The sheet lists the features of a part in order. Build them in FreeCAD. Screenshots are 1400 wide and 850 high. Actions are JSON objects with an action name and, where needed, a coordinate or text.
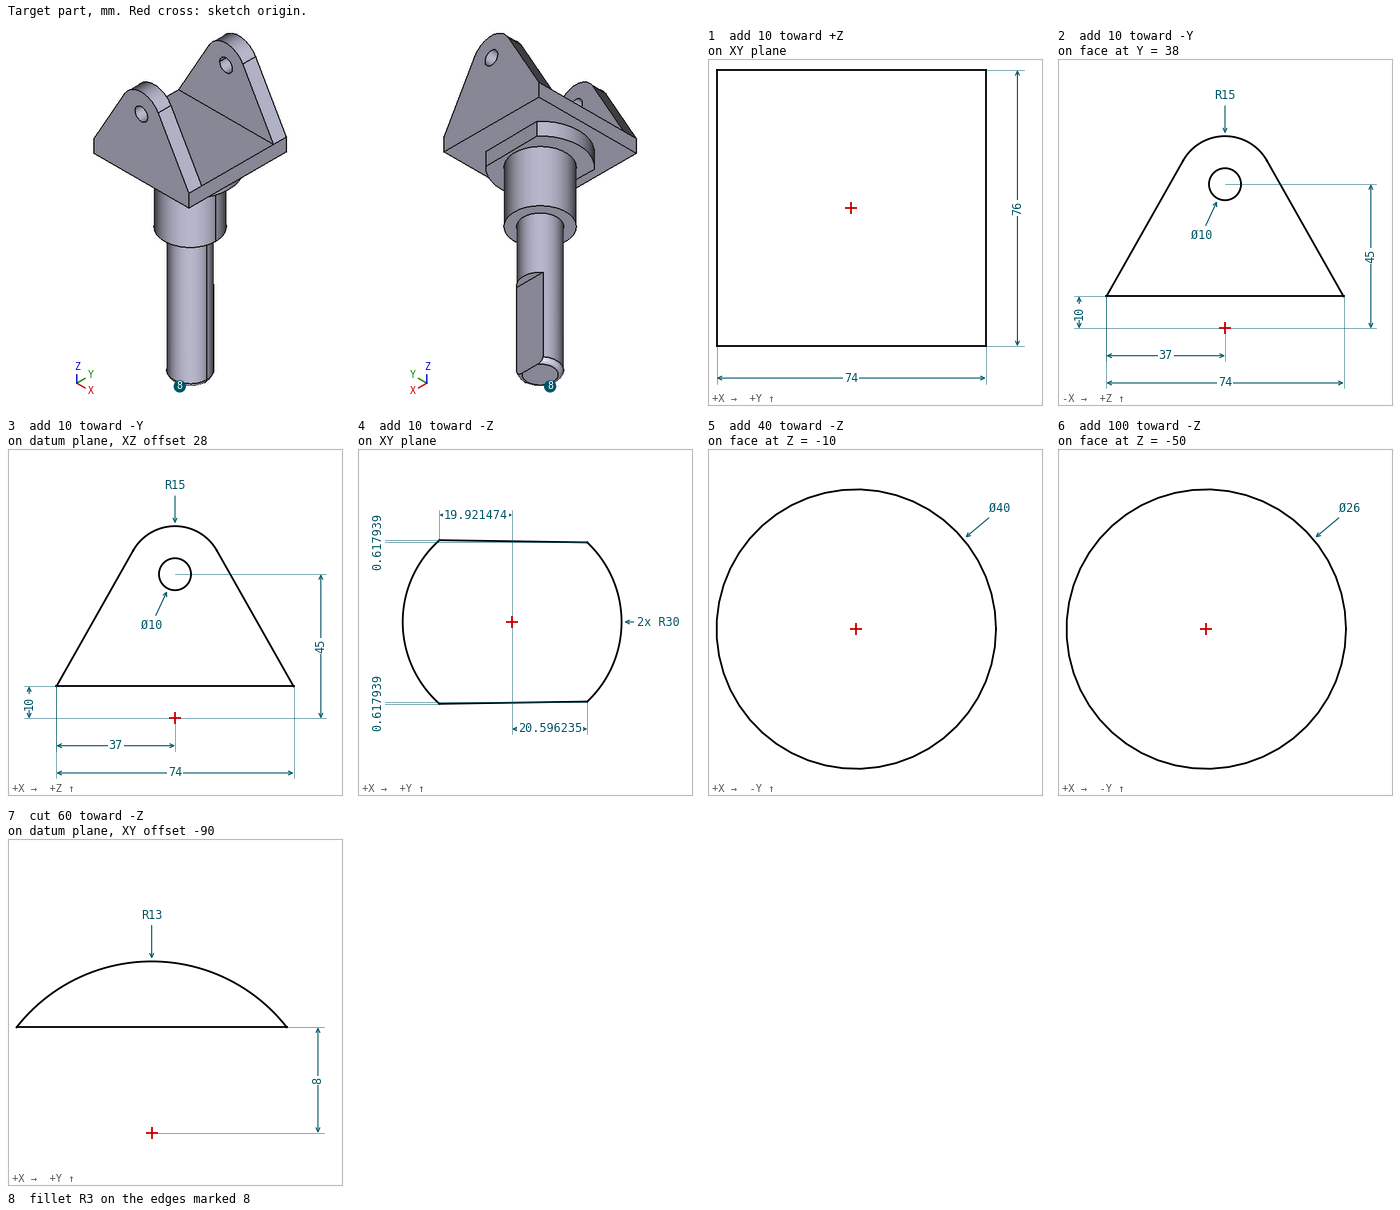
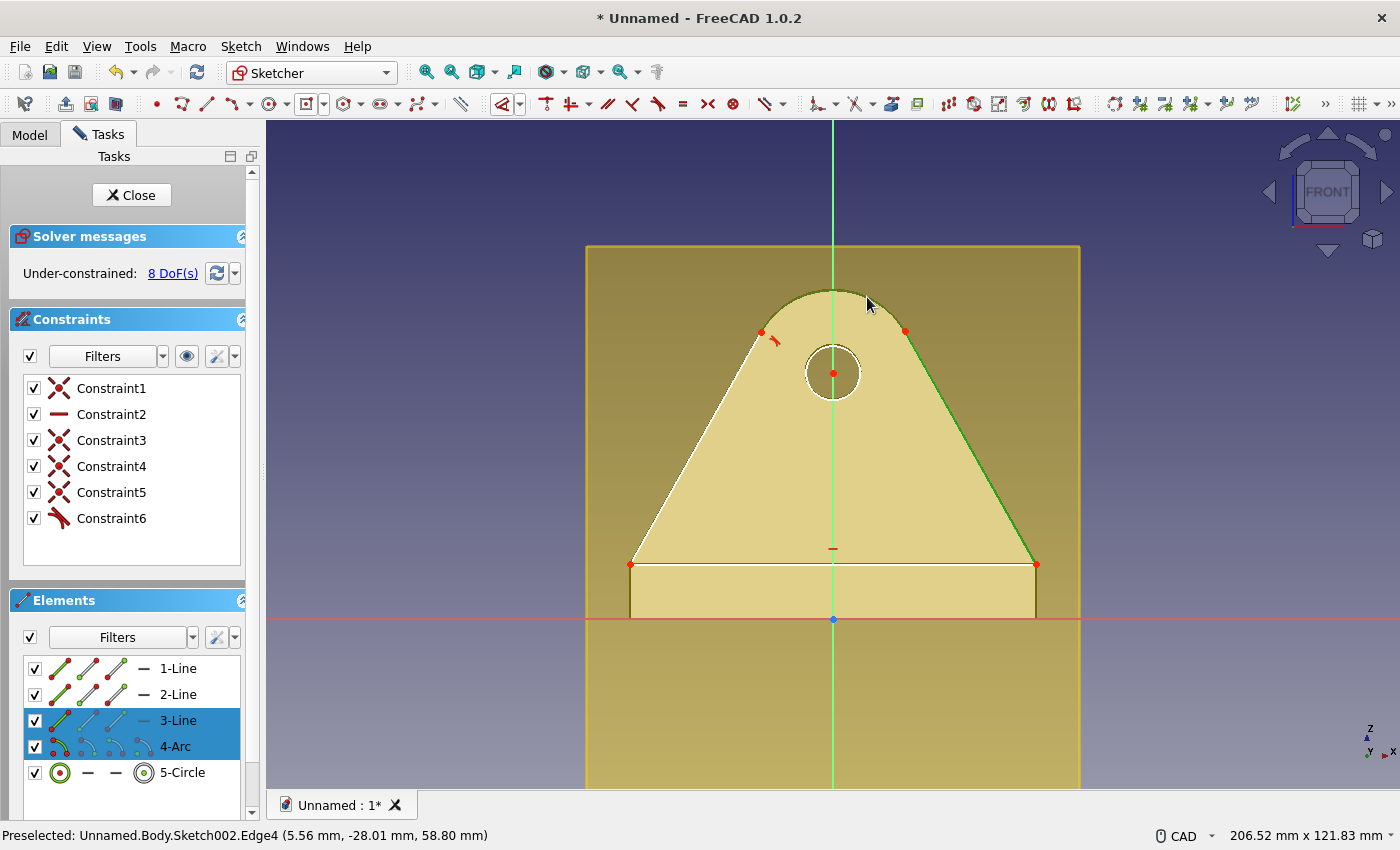
{"action": "left_click", "coordinate": [658, 104]}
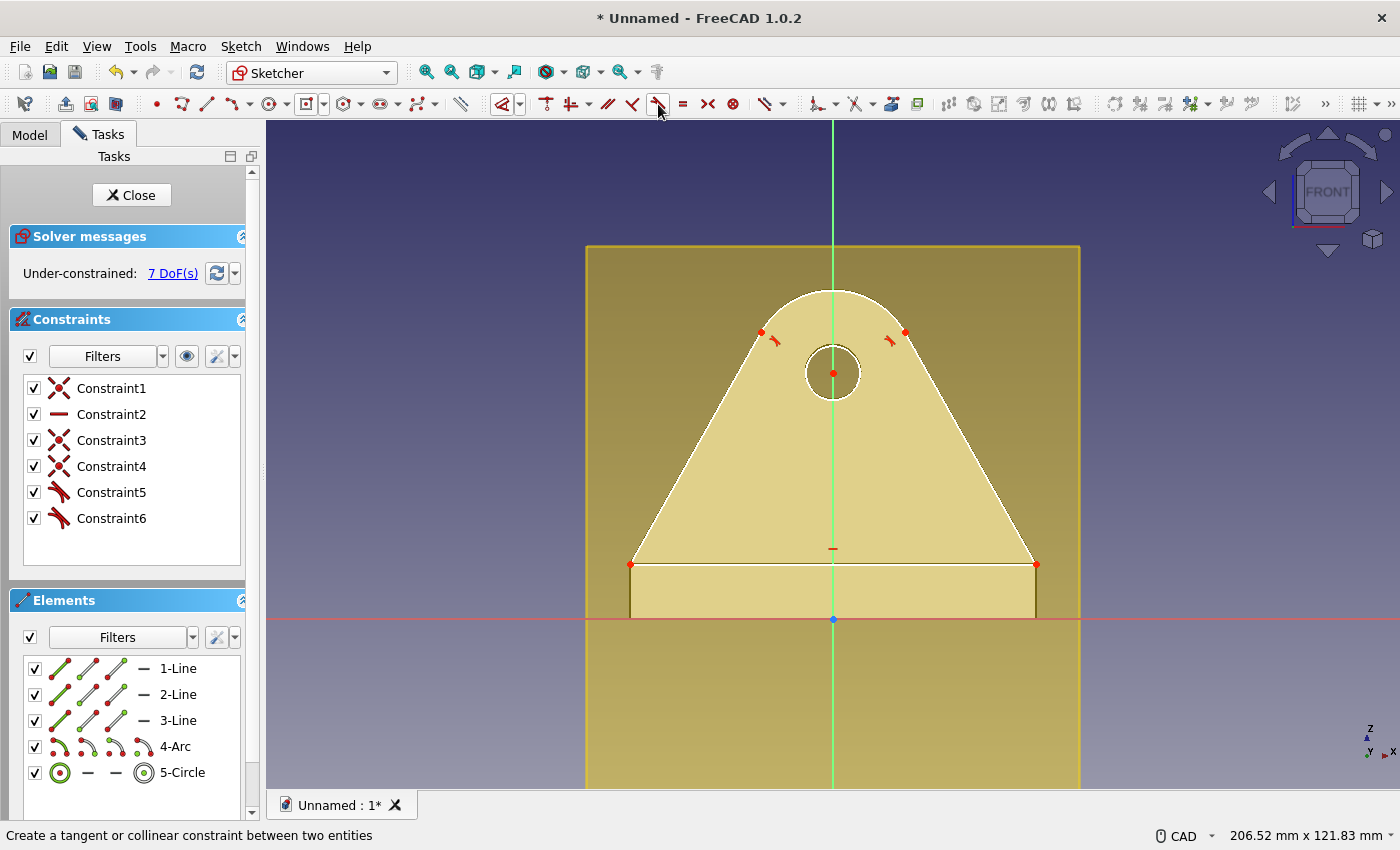
{"action": "left_click", "coordinate": [833, 373]}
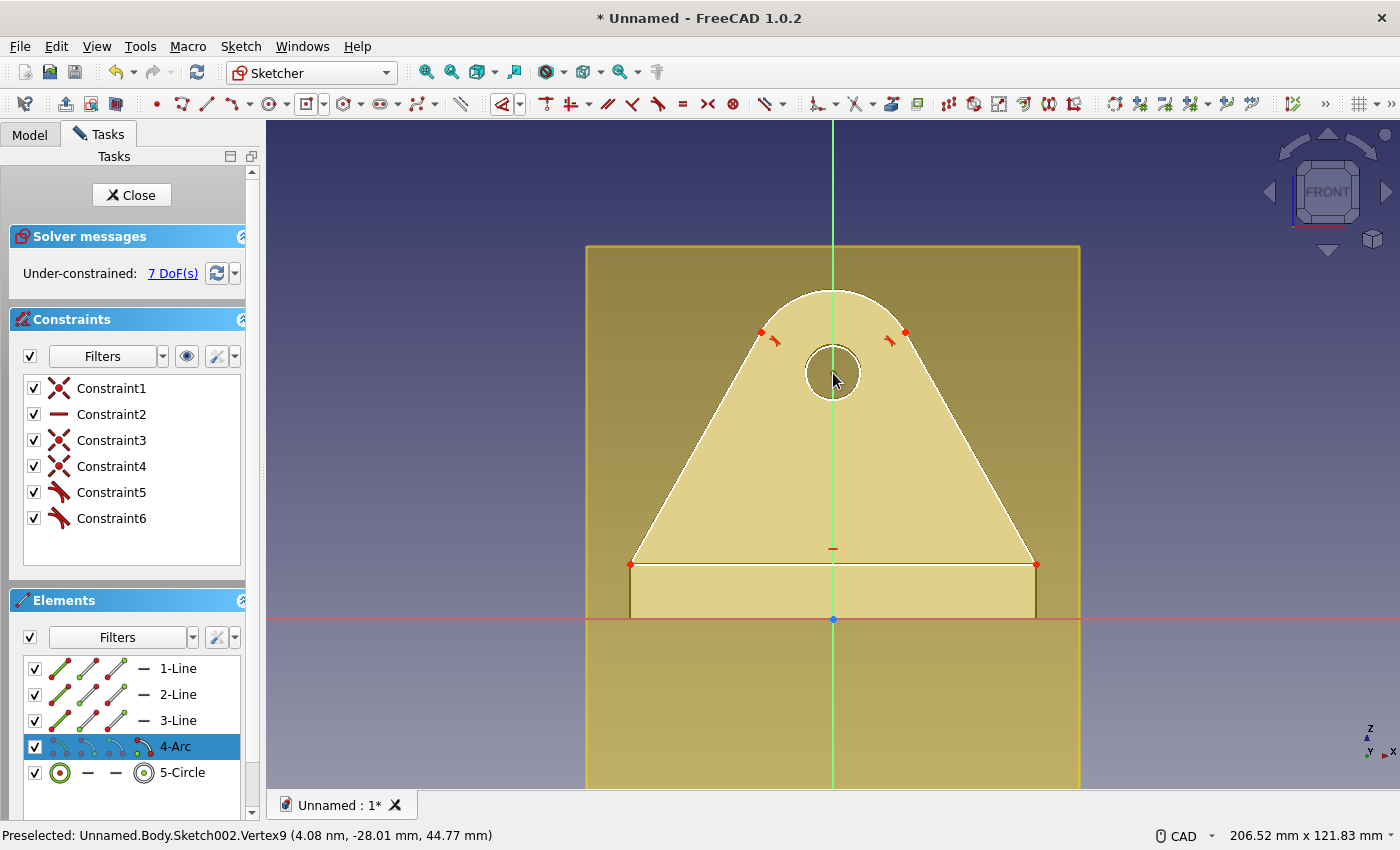
{"action": "left_click", "coordinate": [833, 717]}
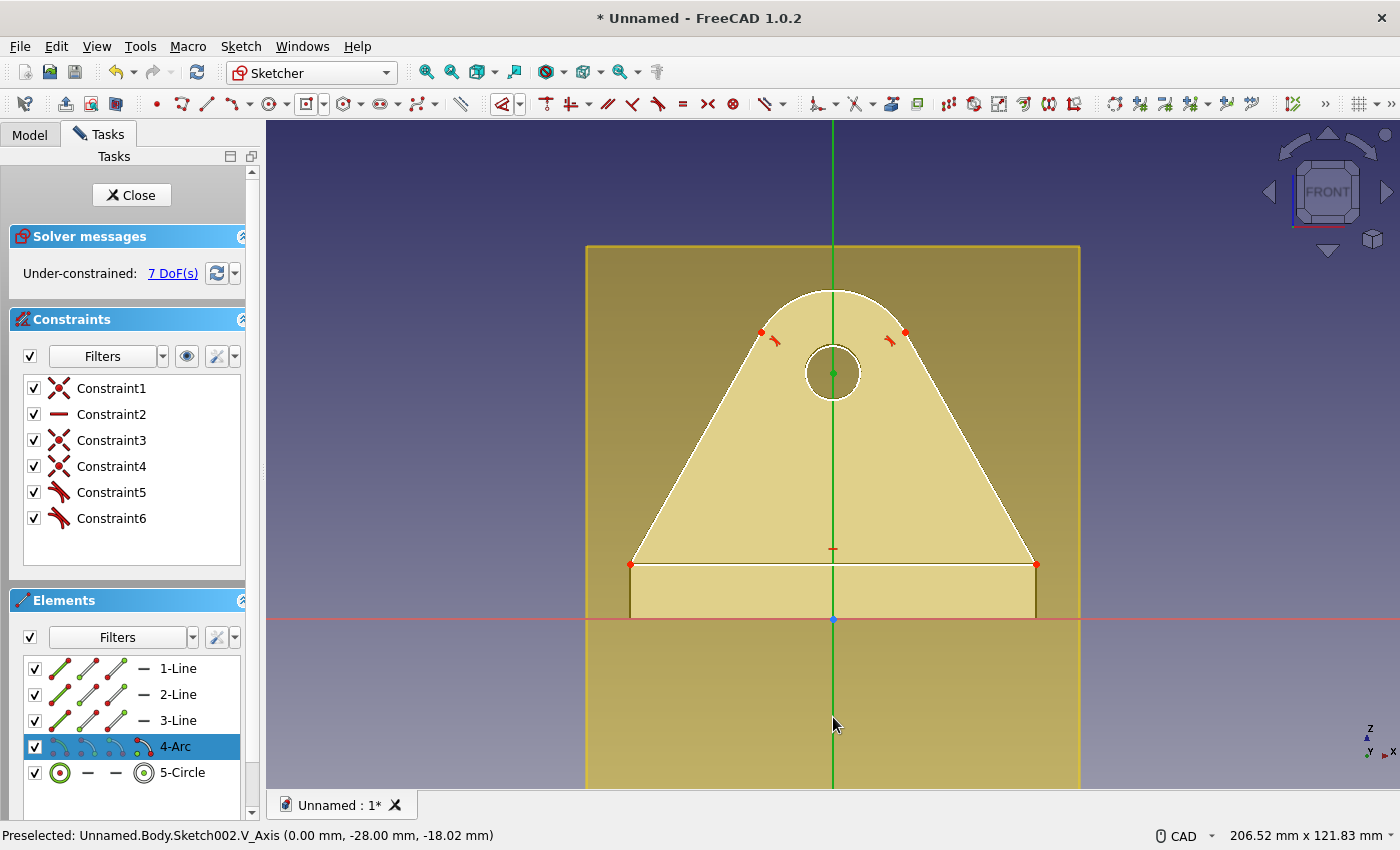
{"action": "left_click", "coordinate": [546, 104]}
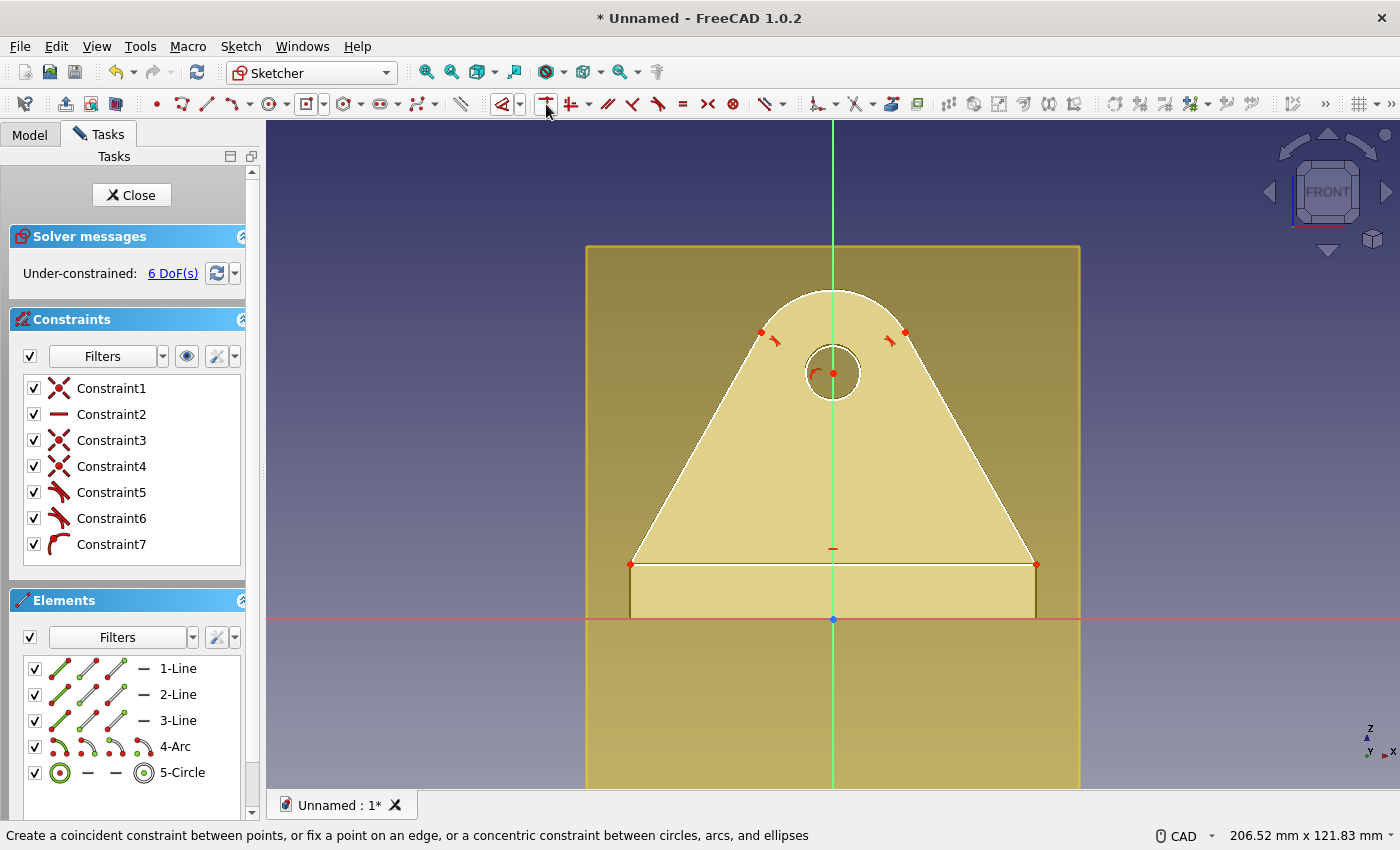
{"action": "left_click", "coordinate": [867, 298]}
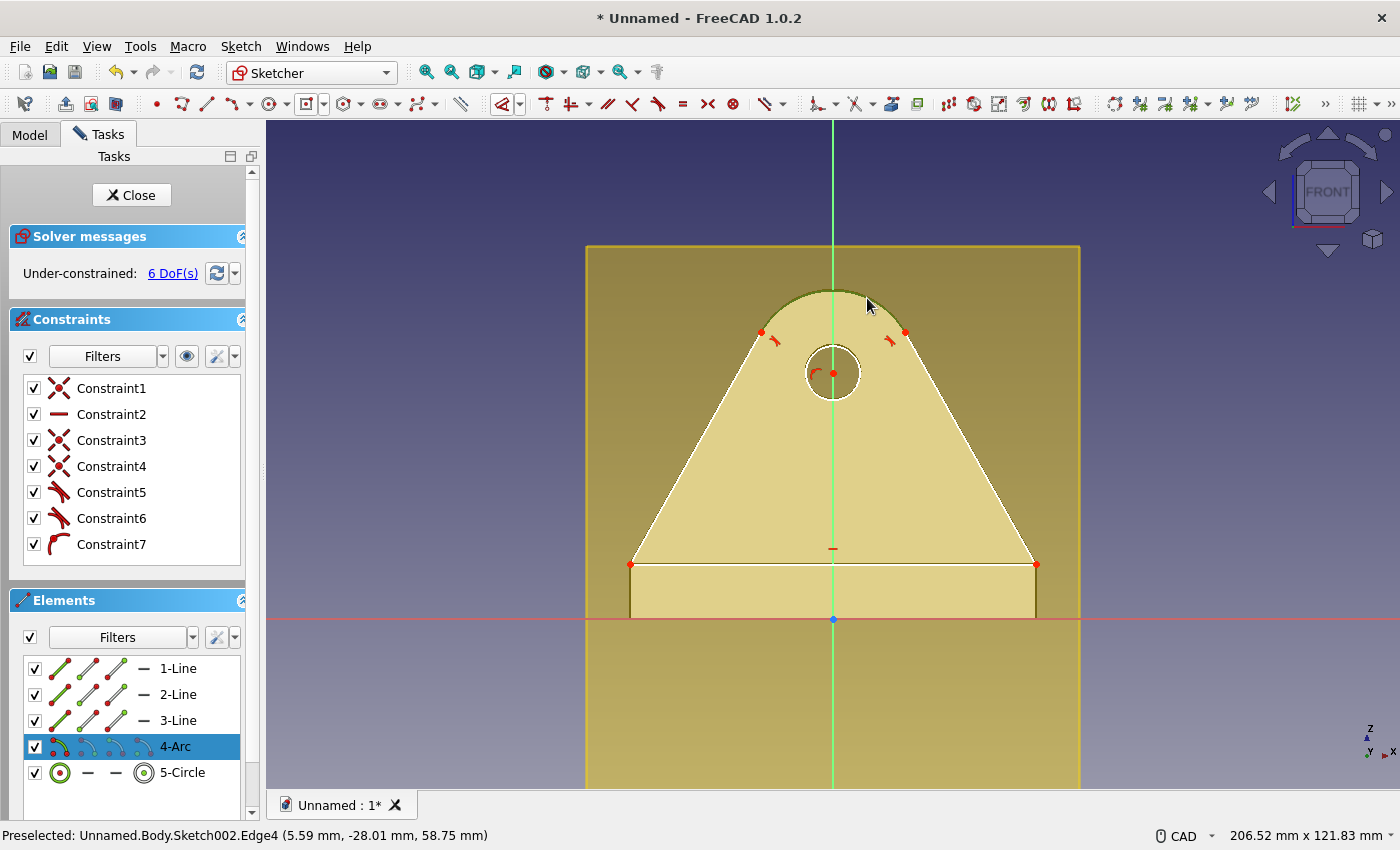
{"action": "left_click", "coordinate": [520, 104]}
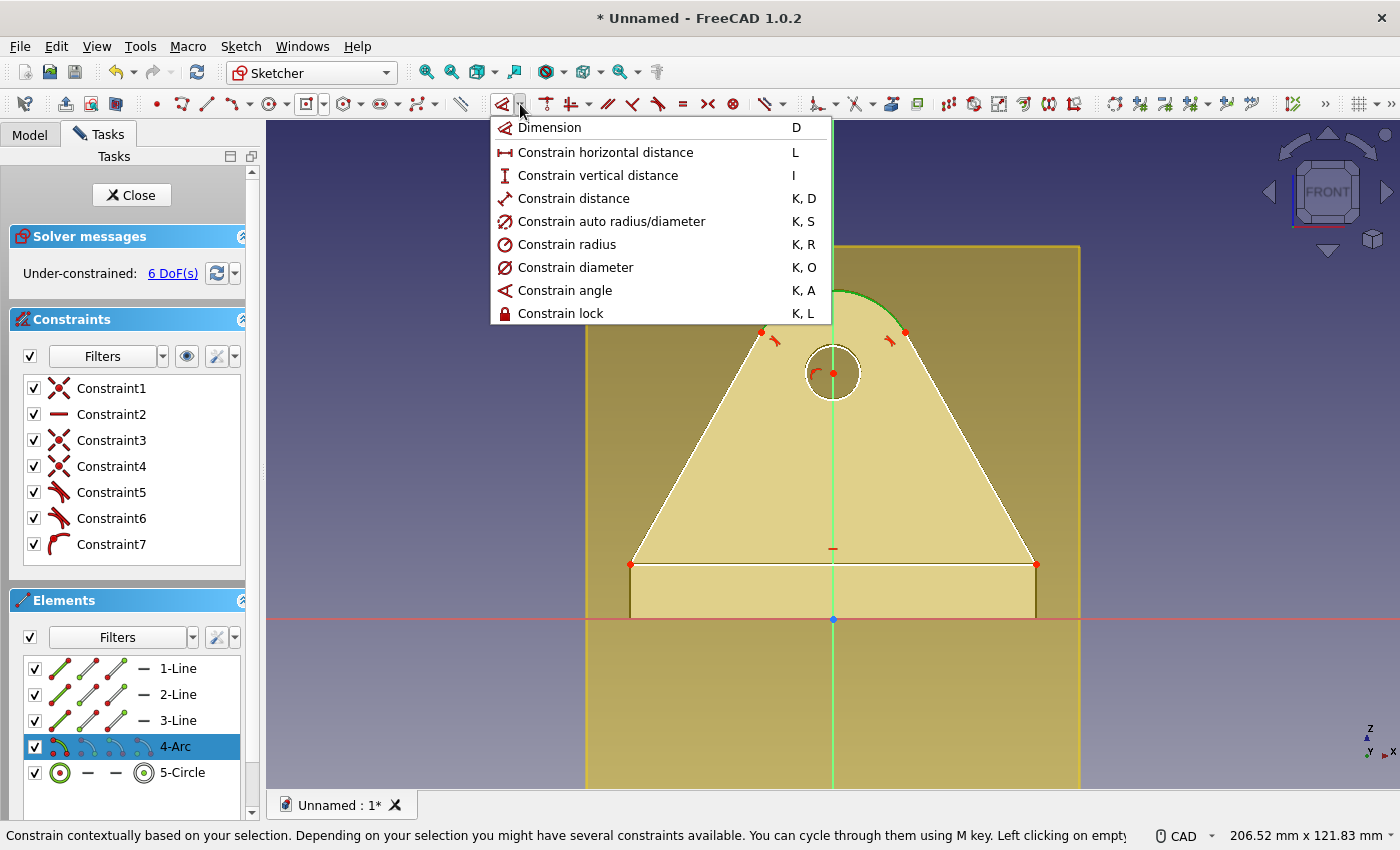
{"action": "left_click", "coordinate": [661, 244]}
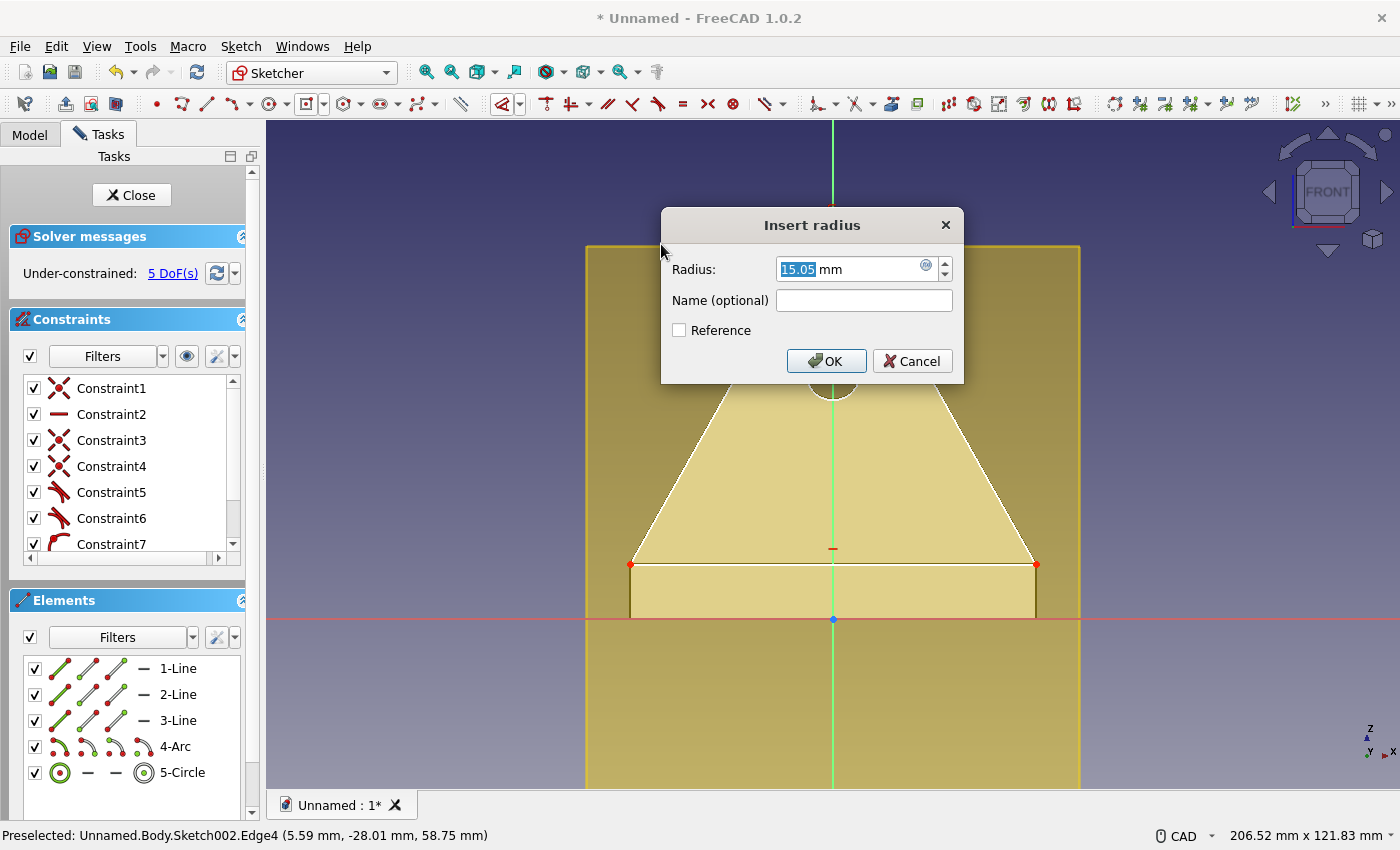
{"action": "type", "text": "15"}
{"action": "key", "text": "Return"}